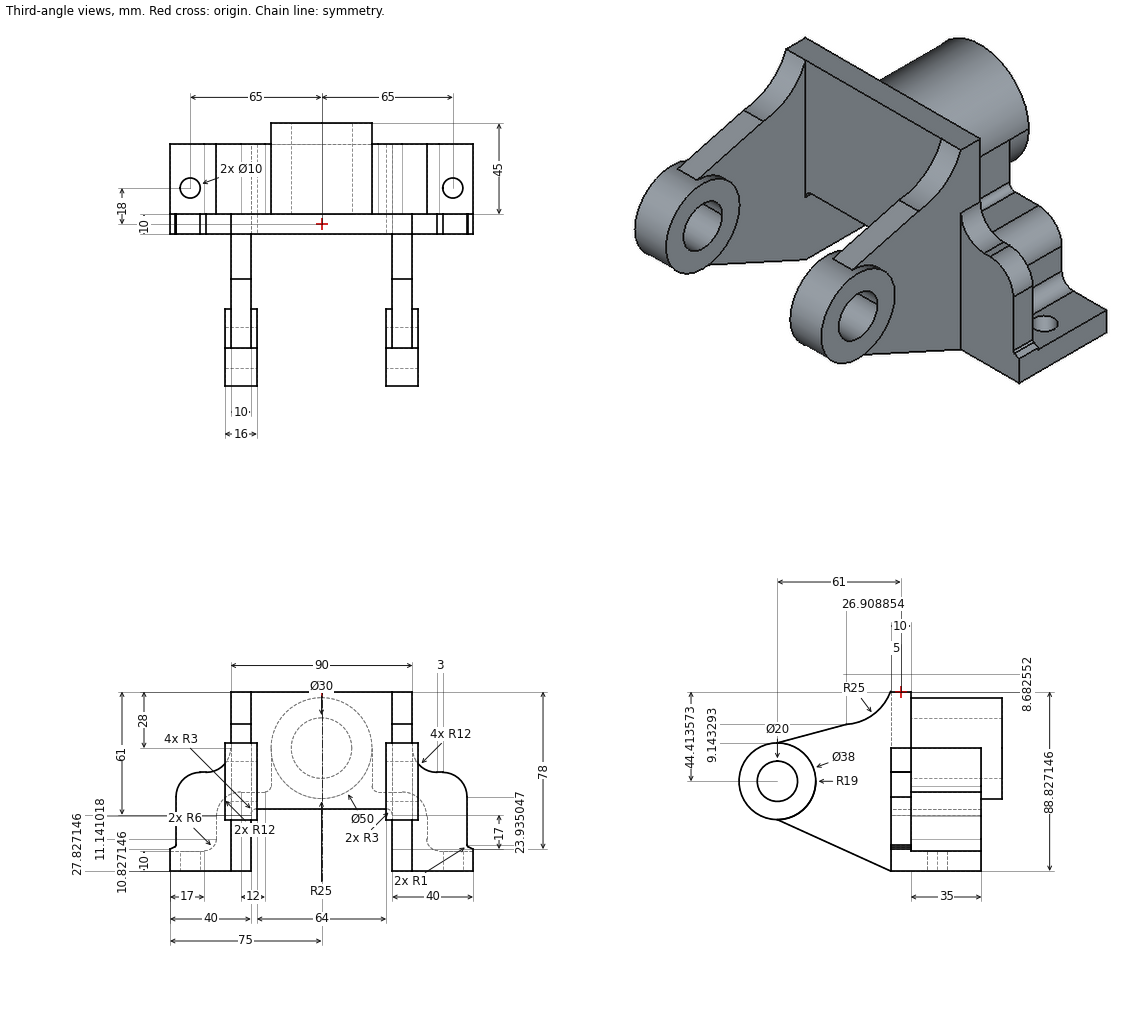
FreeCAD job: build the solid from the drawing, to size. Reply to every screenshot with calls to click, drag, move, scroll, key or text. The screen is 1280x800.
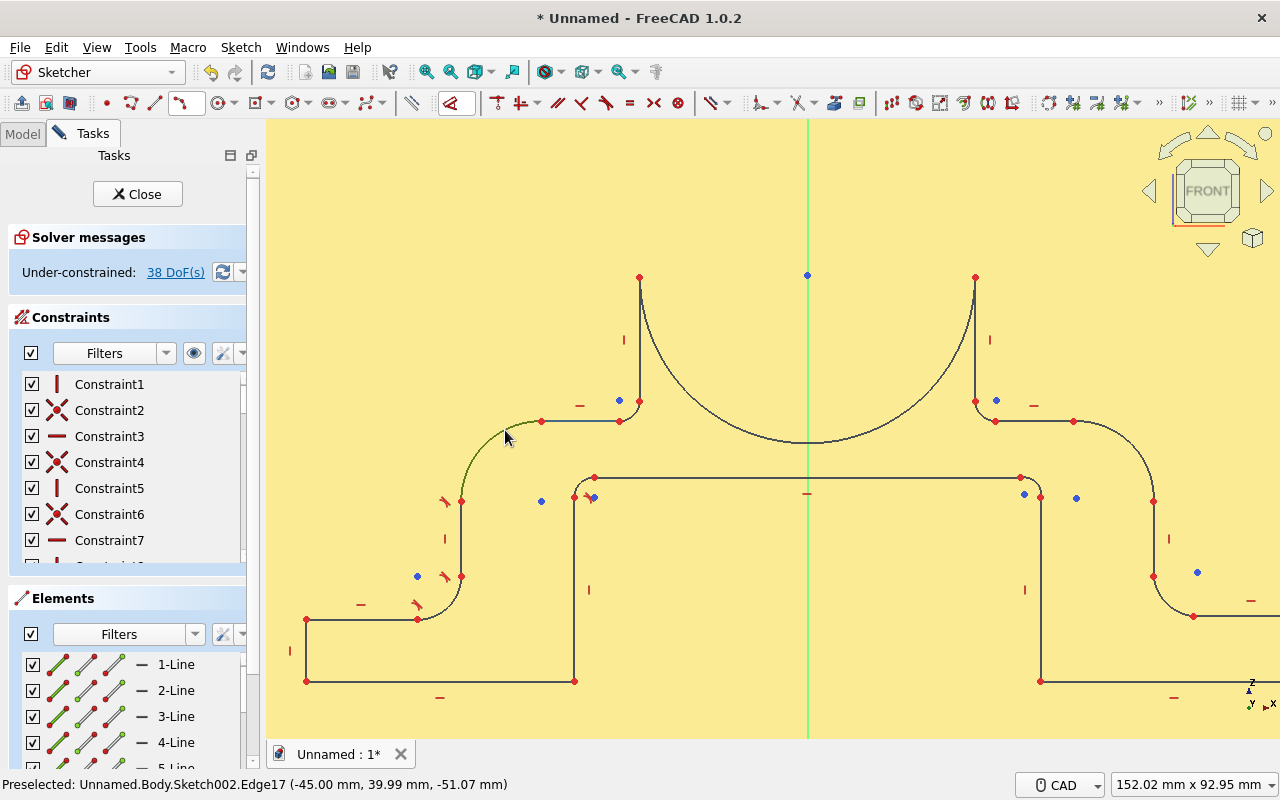
key(t)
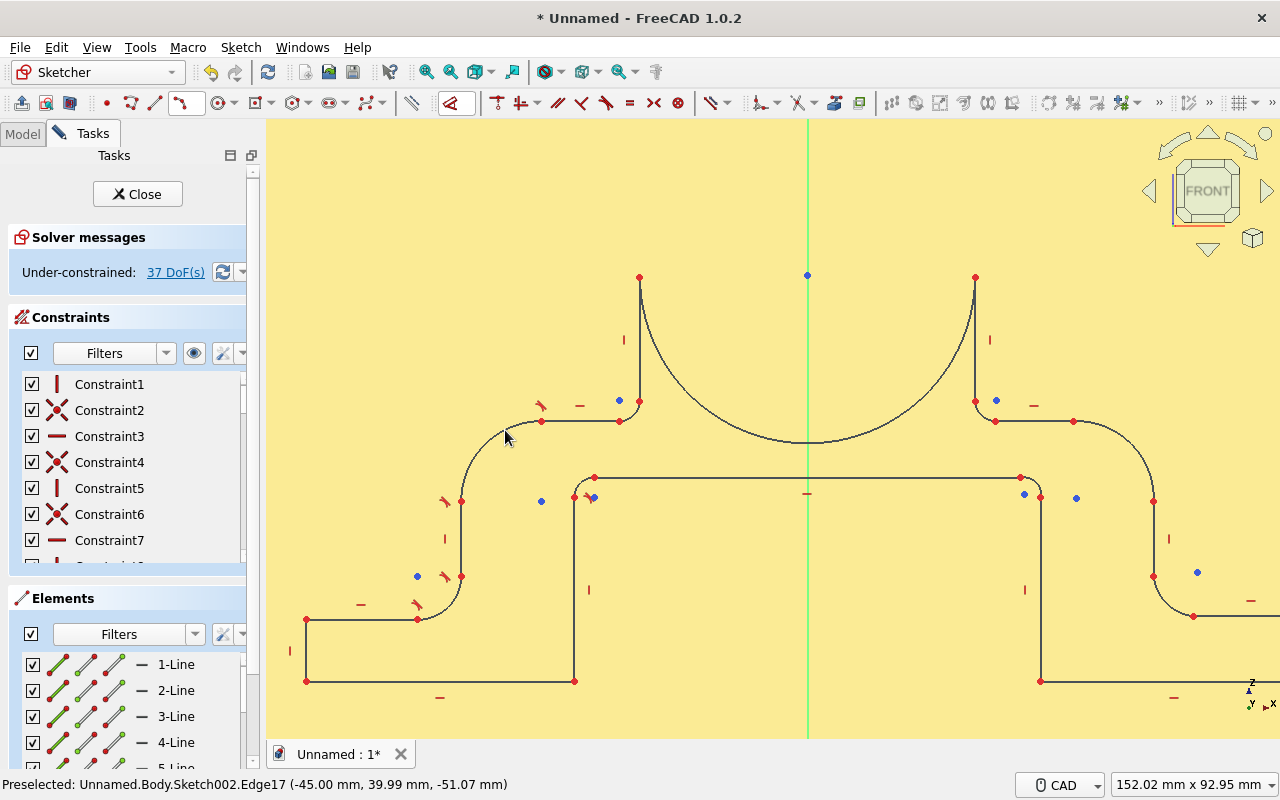
click(565, 421)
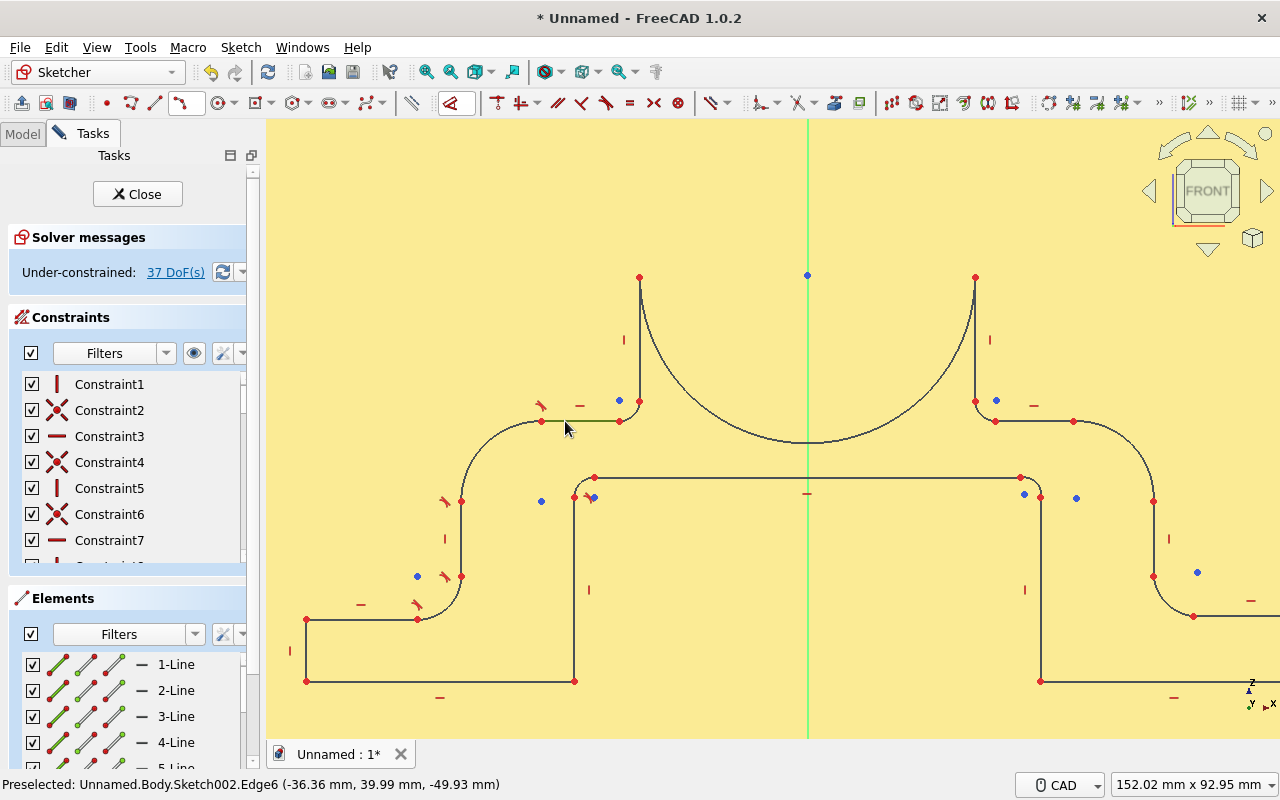
scroll(629, 419, up, 2)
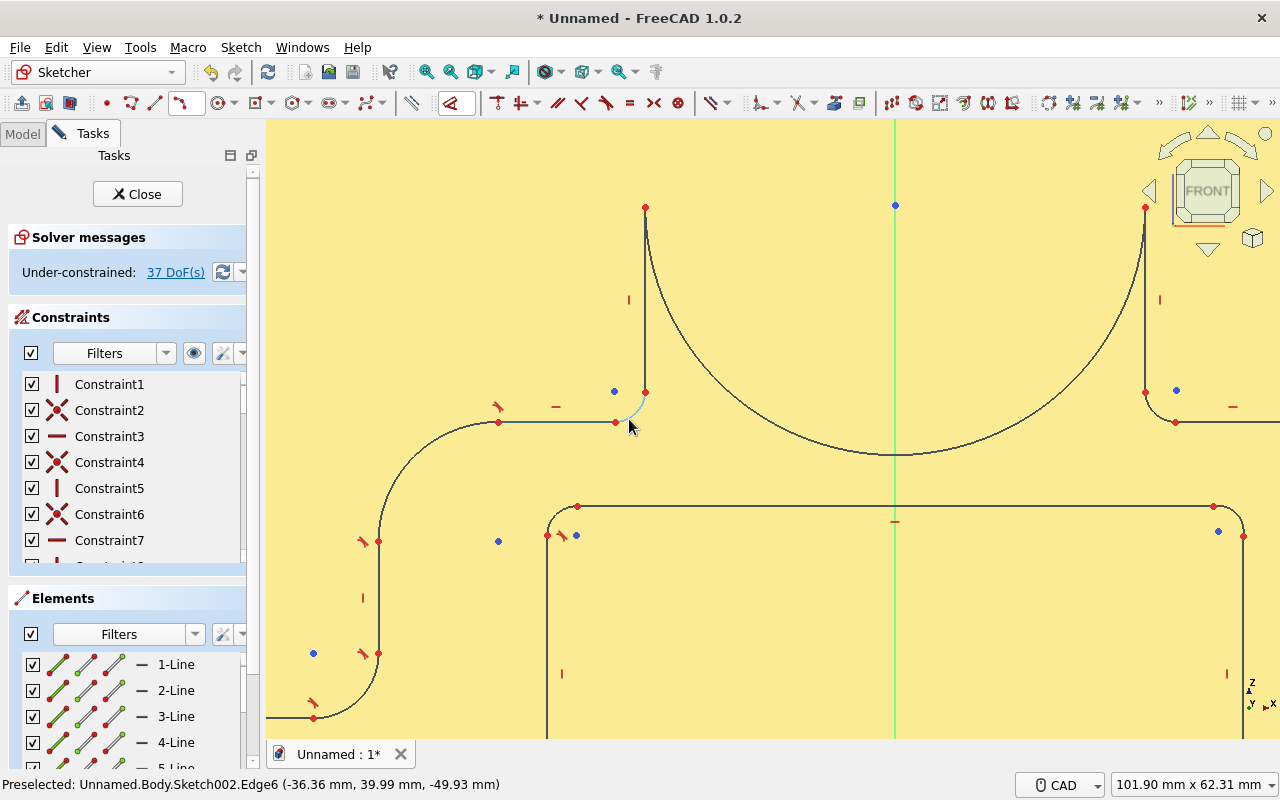
click(629, 418)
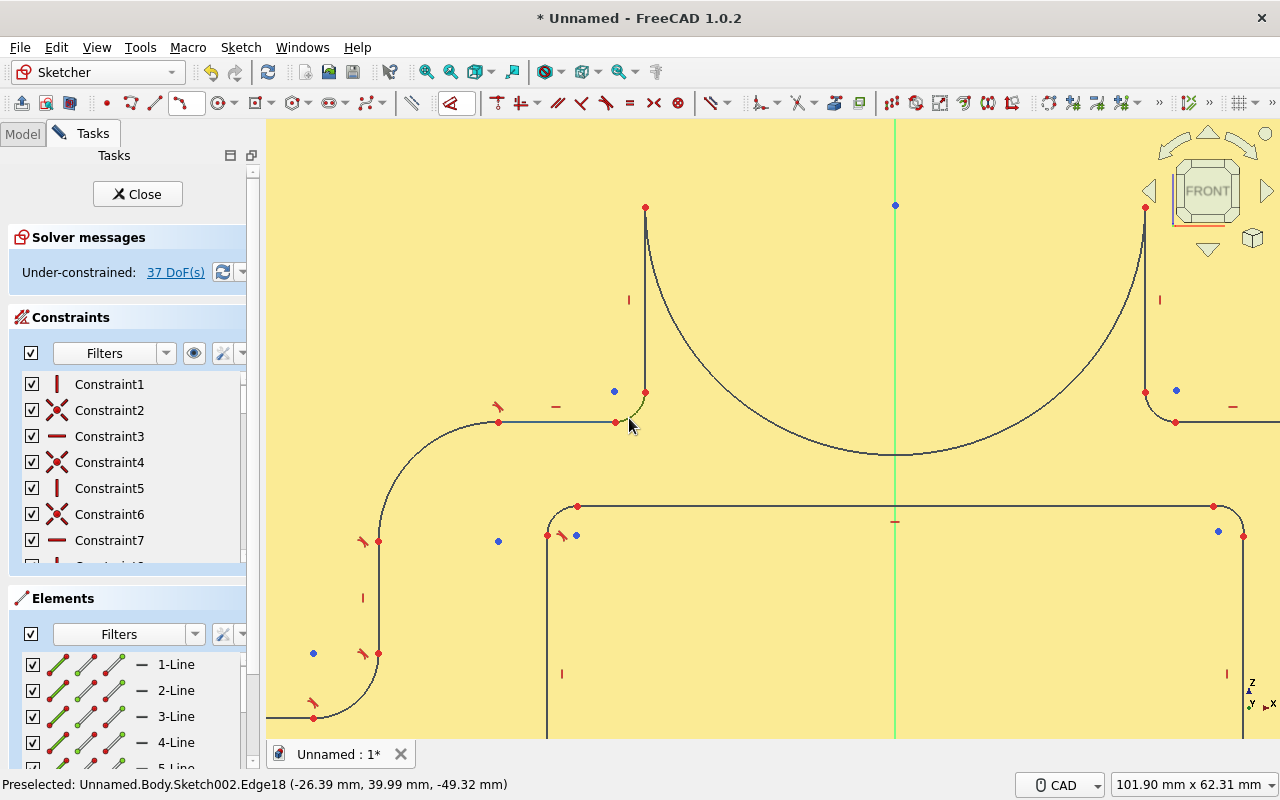
click(606, 104)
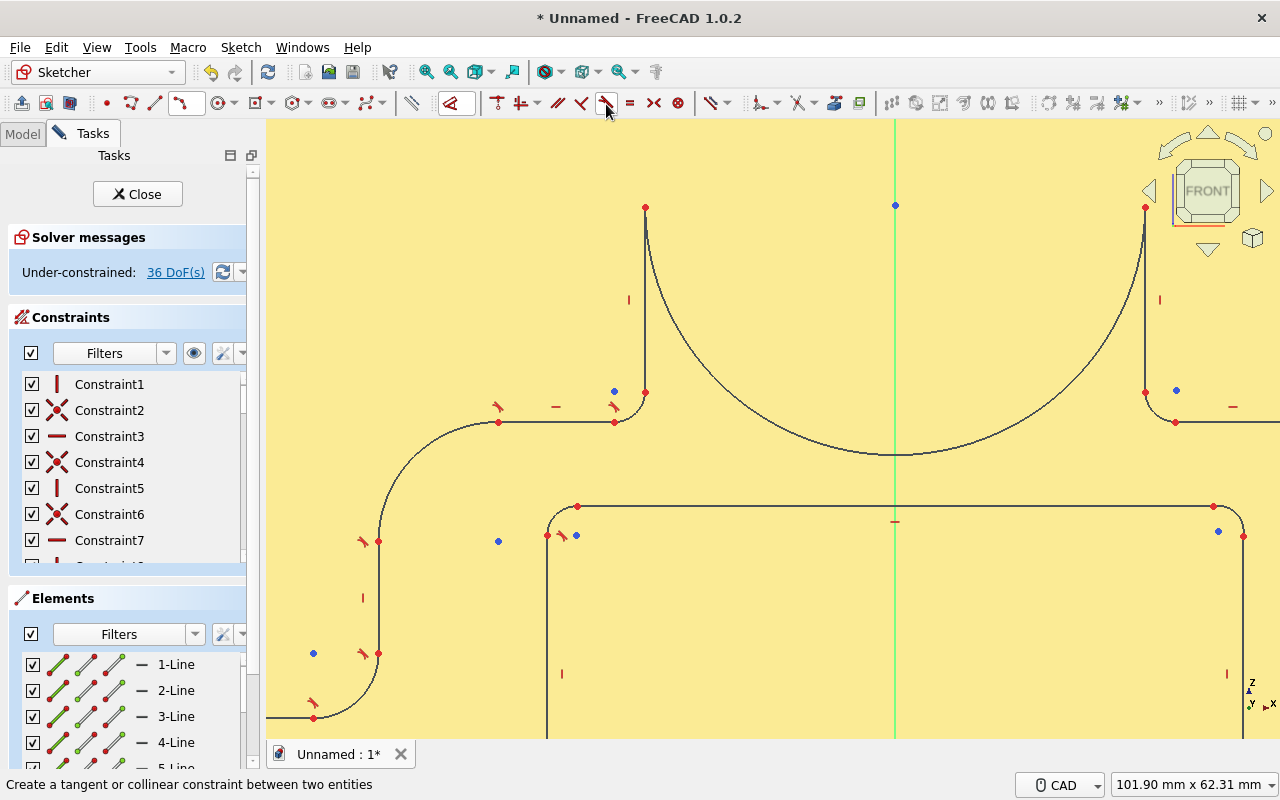
click(645, 337)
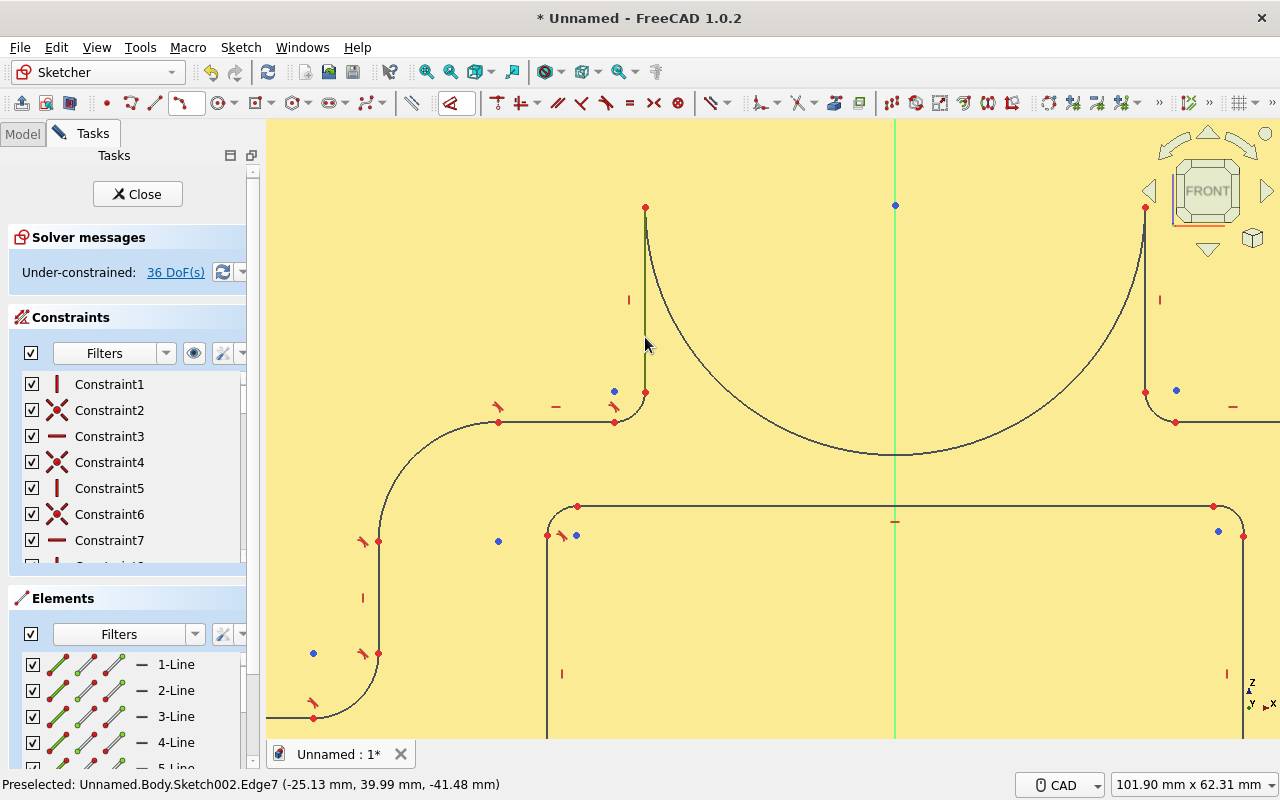
click(628, 419)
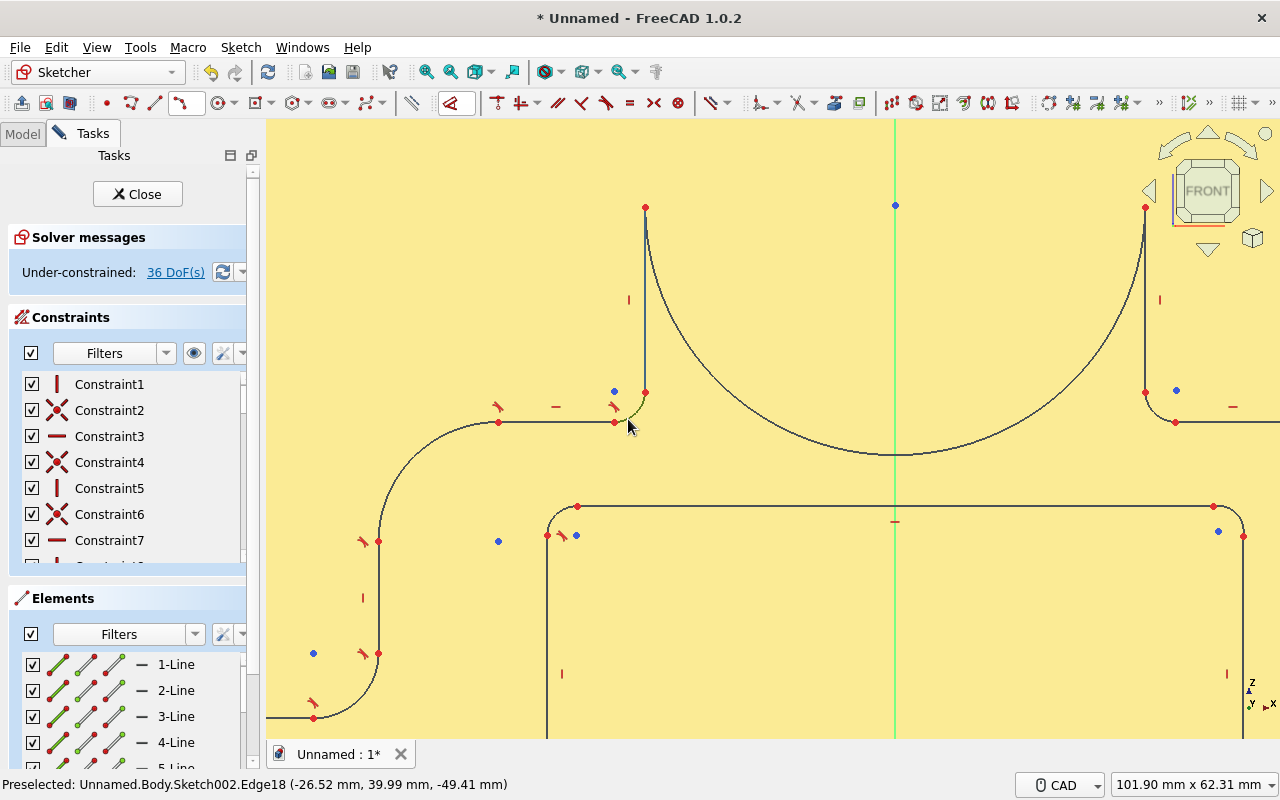
key(t)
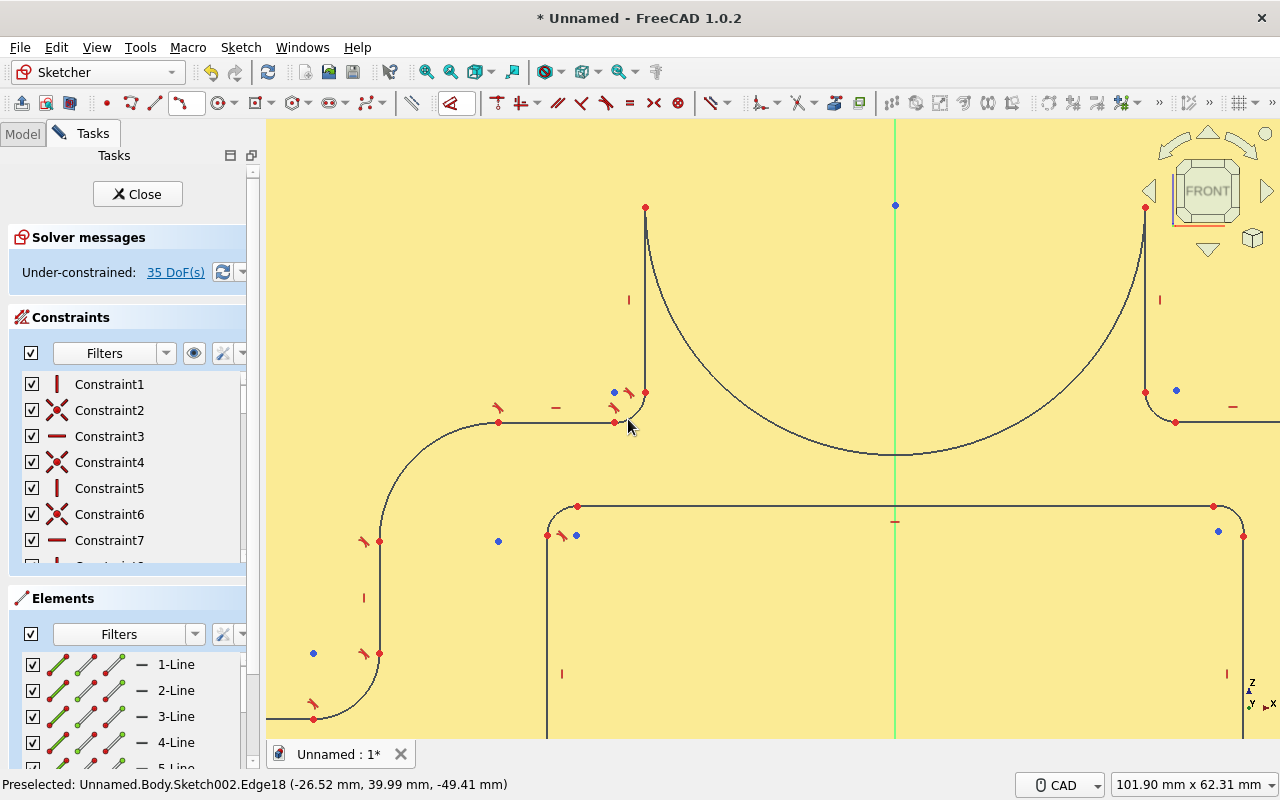
click(645, 337)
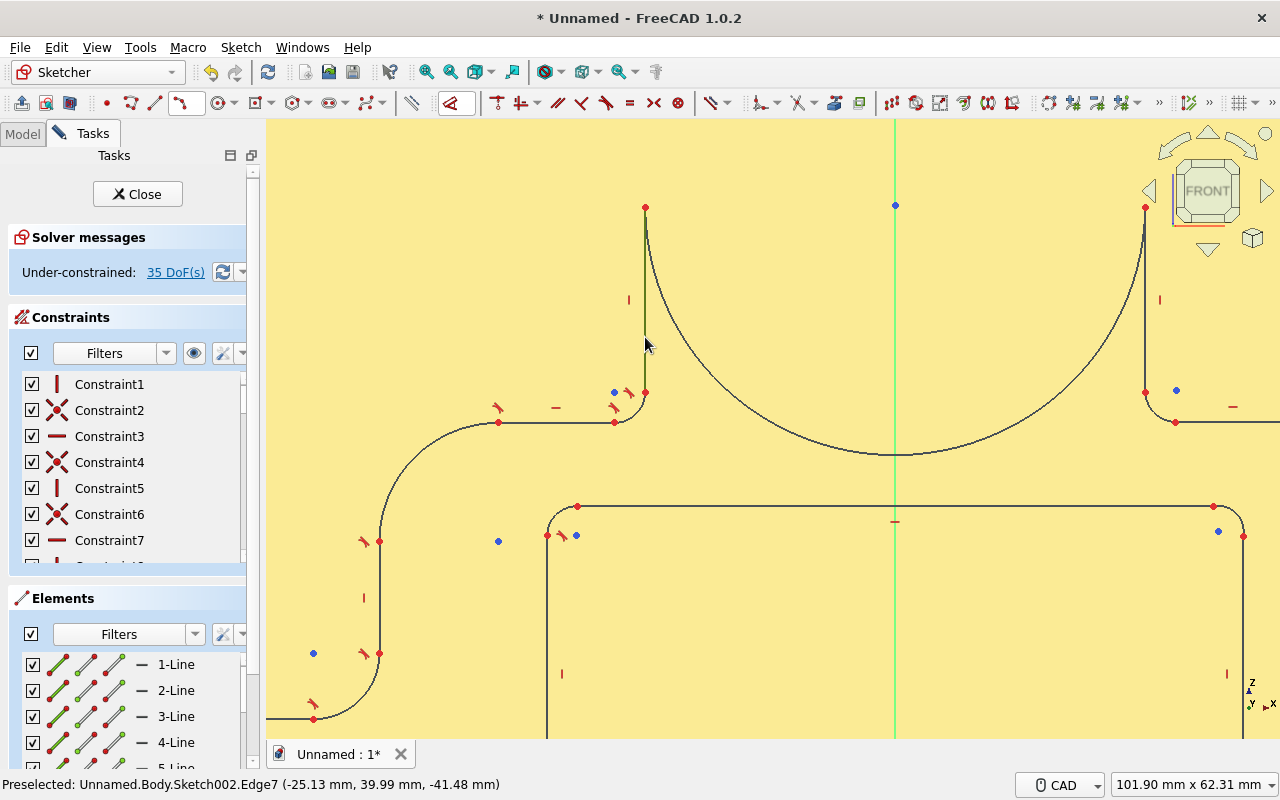
click(749, 408)